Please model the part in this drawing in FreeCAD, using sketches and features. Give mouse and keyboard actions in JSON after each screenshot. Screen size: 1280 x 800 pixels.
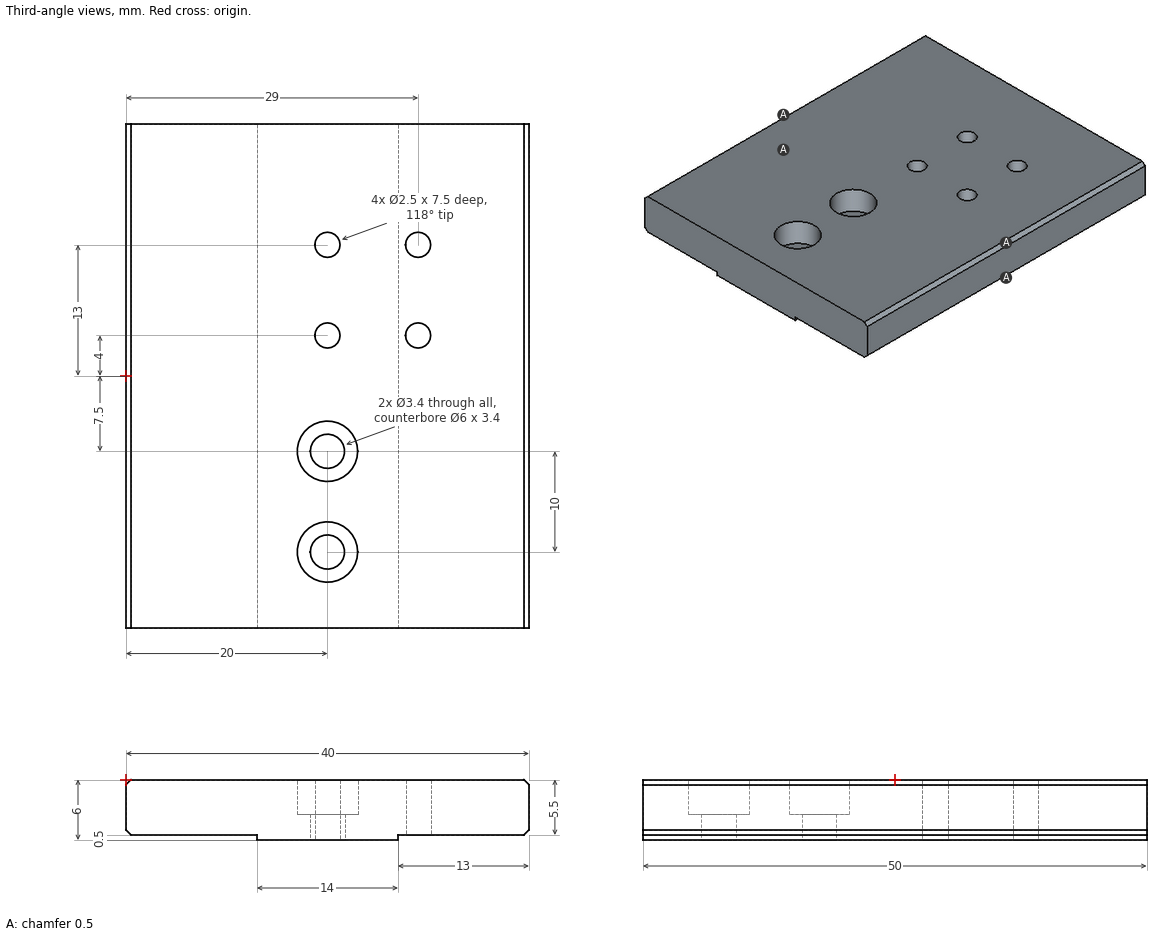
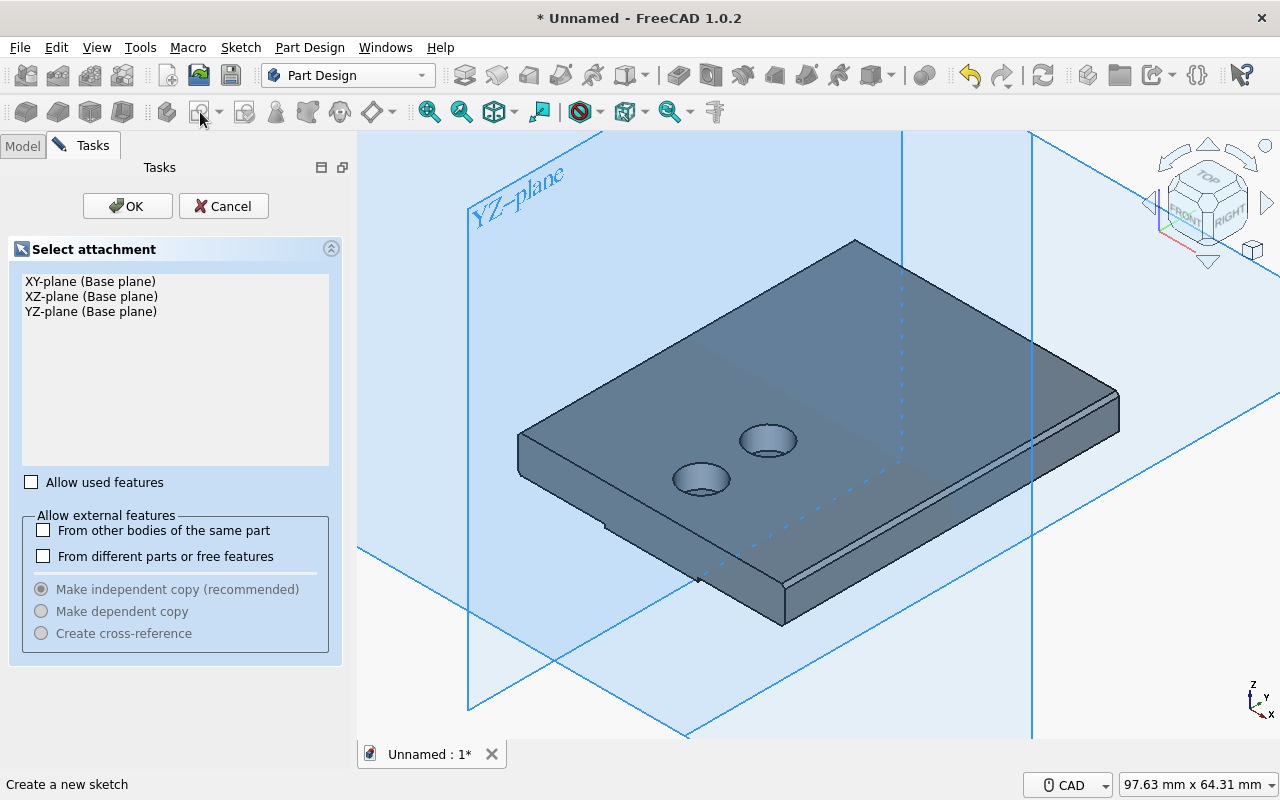
{"action": "left_click", "coordinate": [82, 282]}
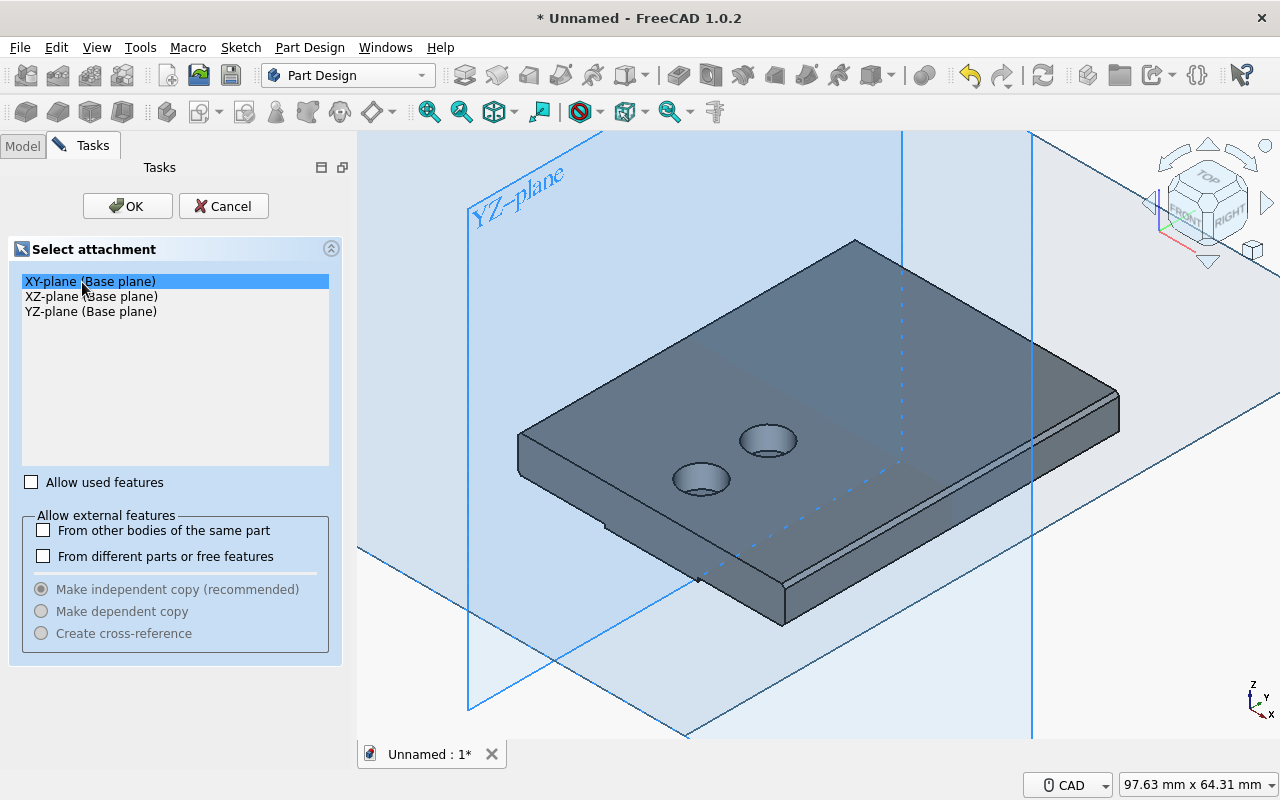
{"action": "left_click", "coordinate": [128, 206]}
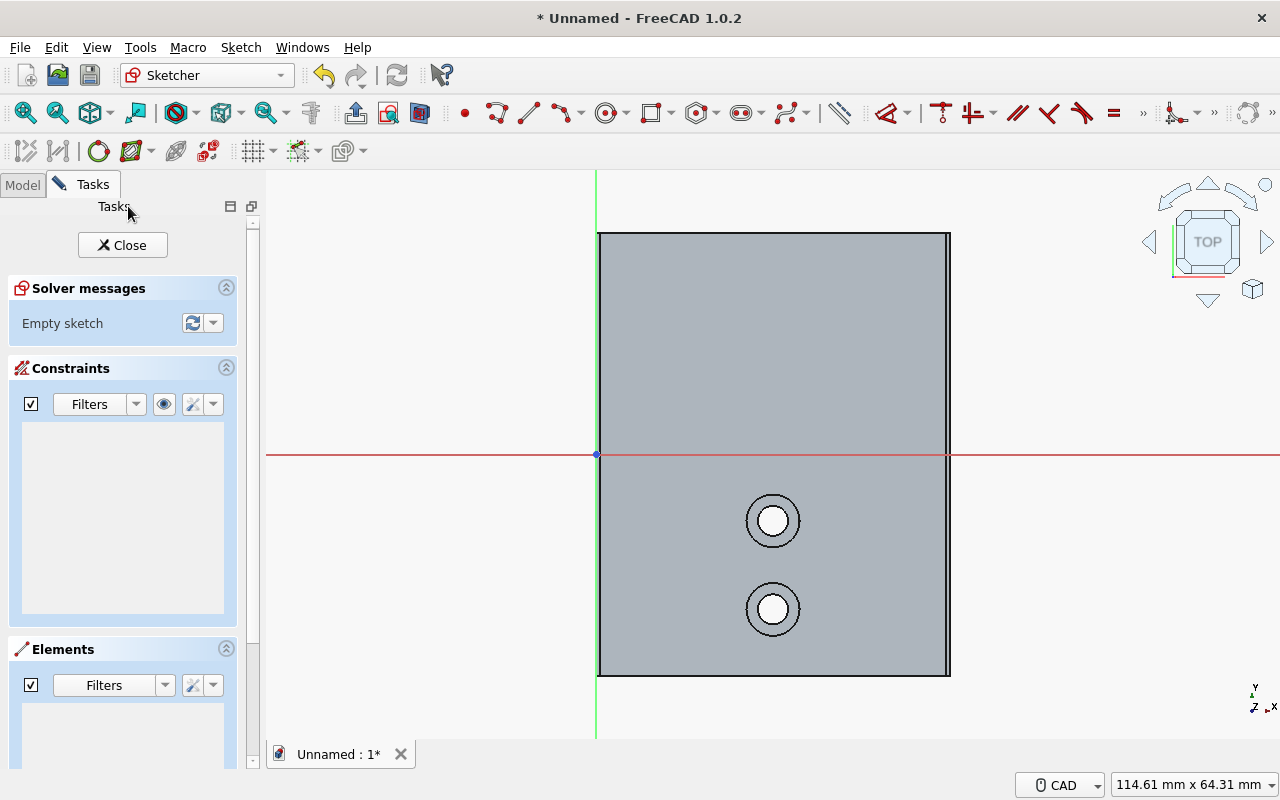
{"action": "scroll", "coordinate": [859, 347], "scroll_direction": "up", "scroll_amount": 6}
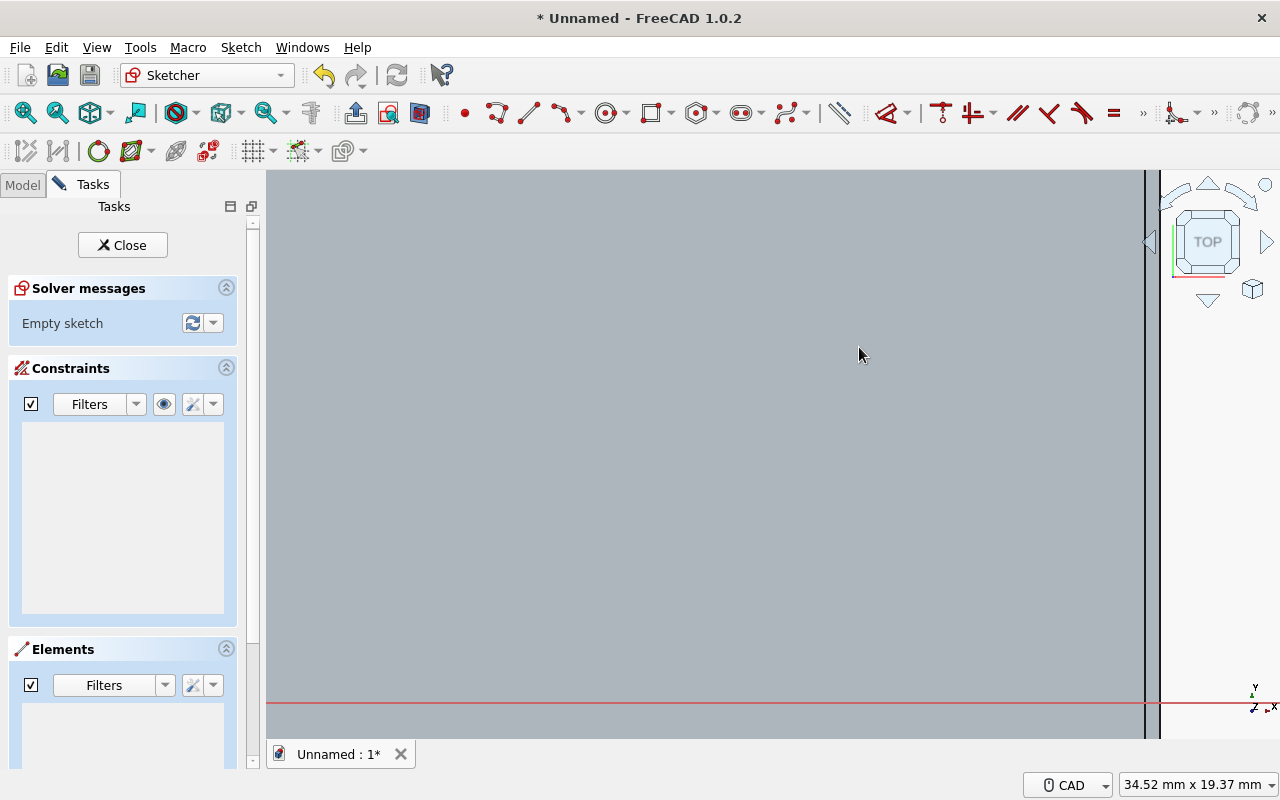
{"action": "left_click", "coordinate": [606, 114]}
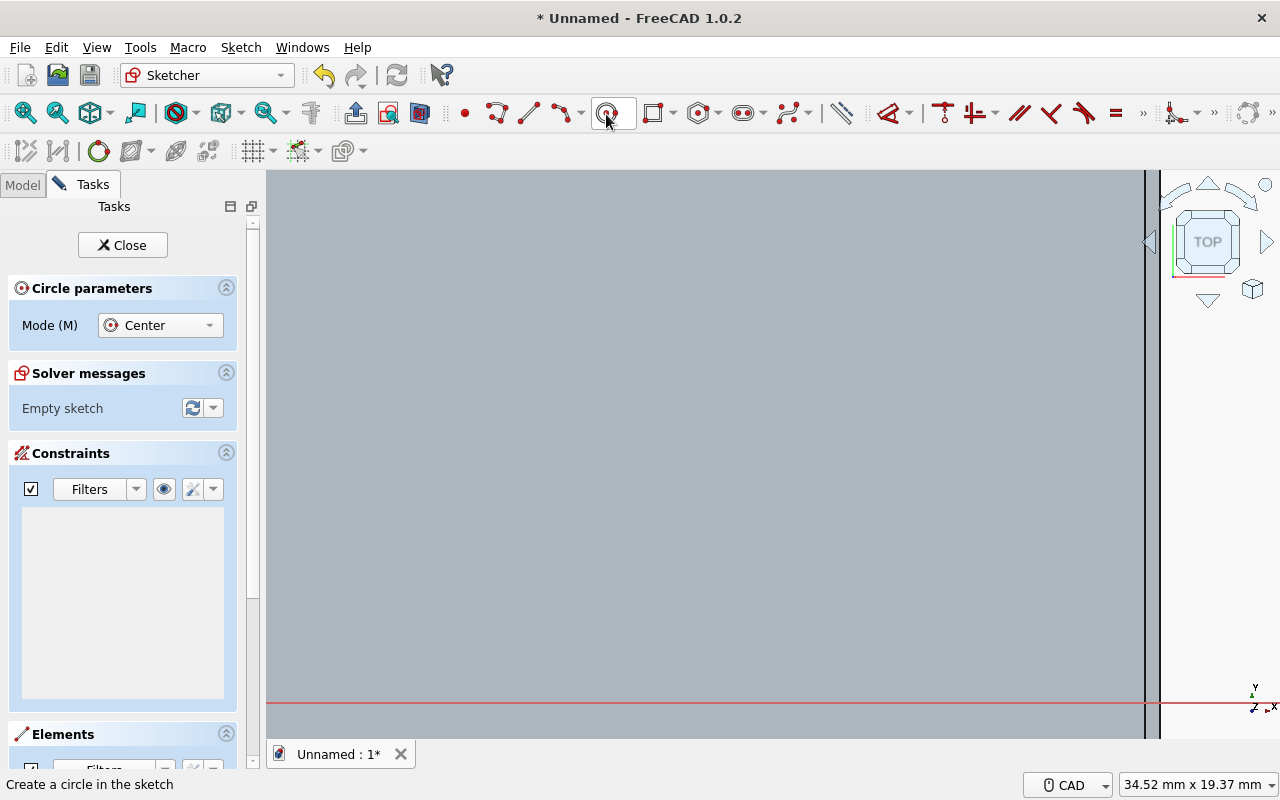
{"action": "left_click", "coordinate": [572, 321]}
{"action": "mouse_move", "coordinate": [598, 295]}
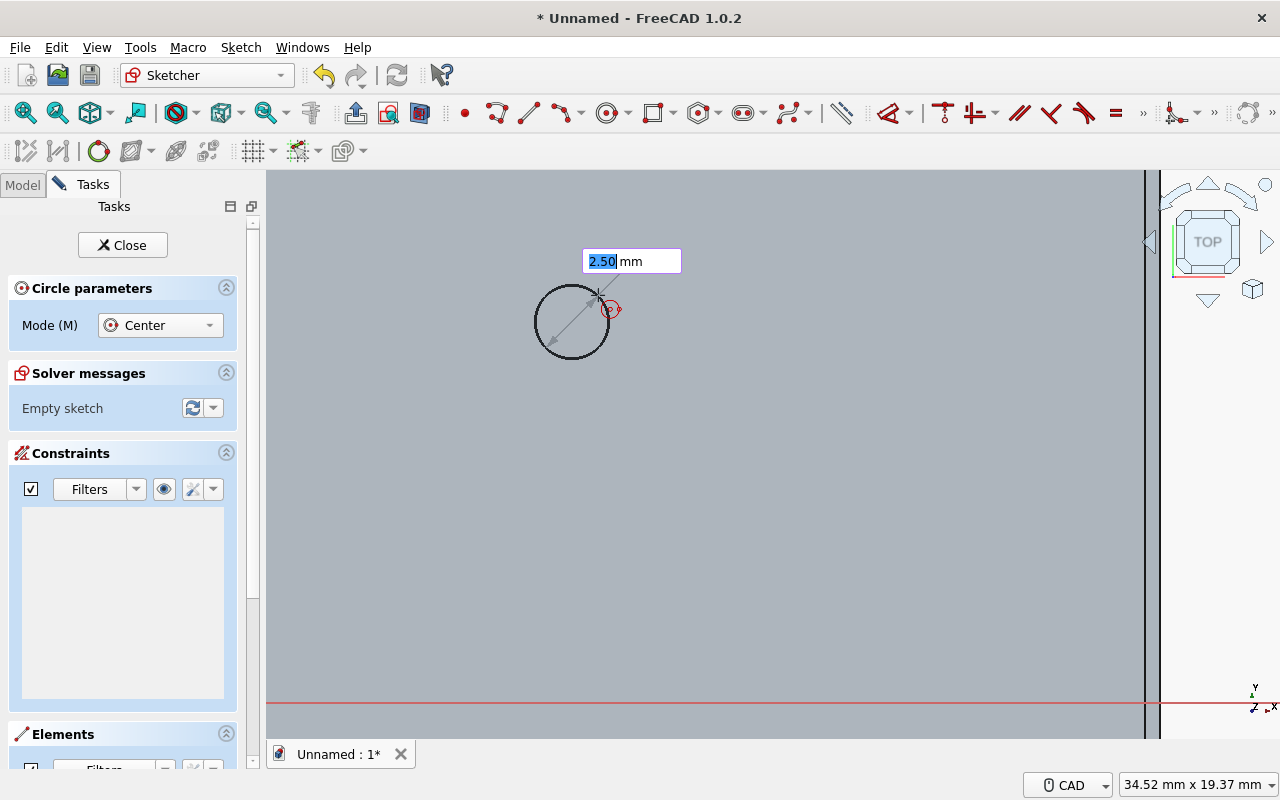
{"action": "type", "text": "2.5"}
{"action": "key", "text": "Return"}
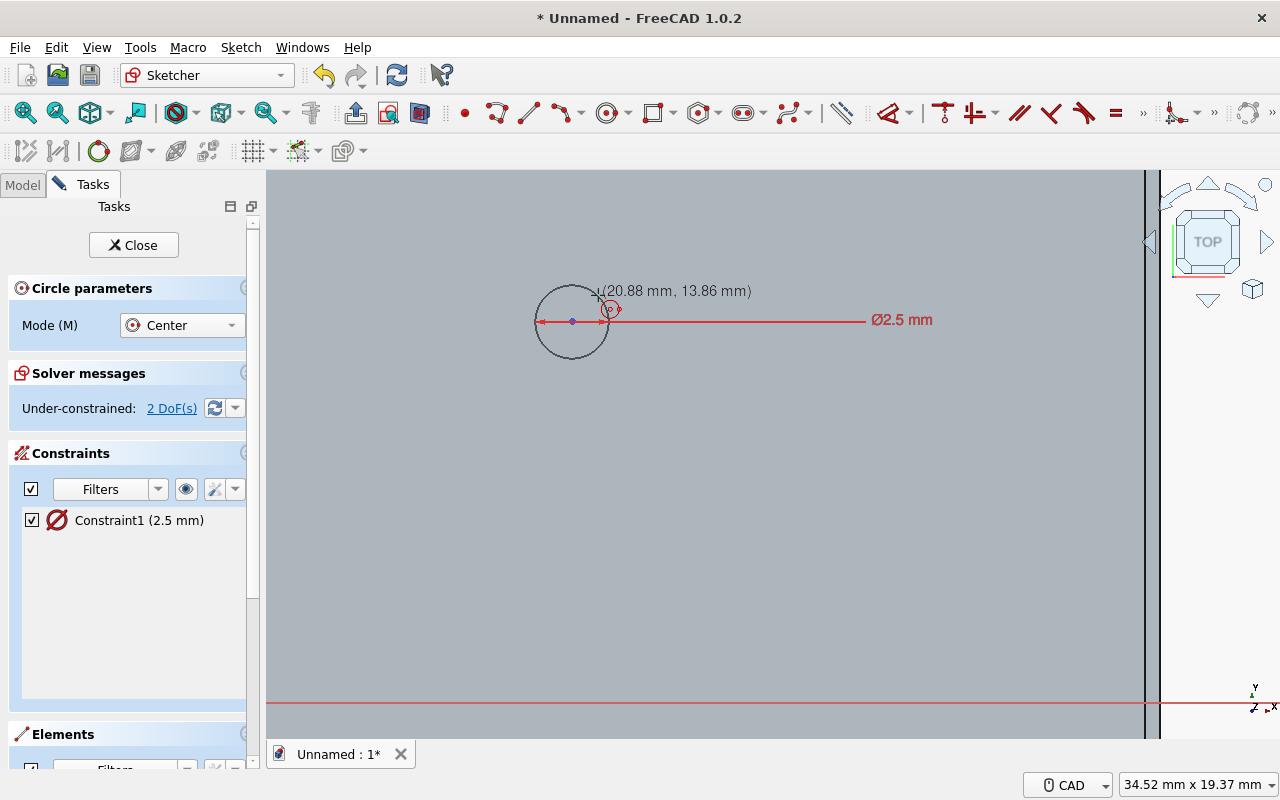
{"action": "left_click", "coordinate": [836, 321]}
{"action": "mouse_move", "coordinate": [862, 295]}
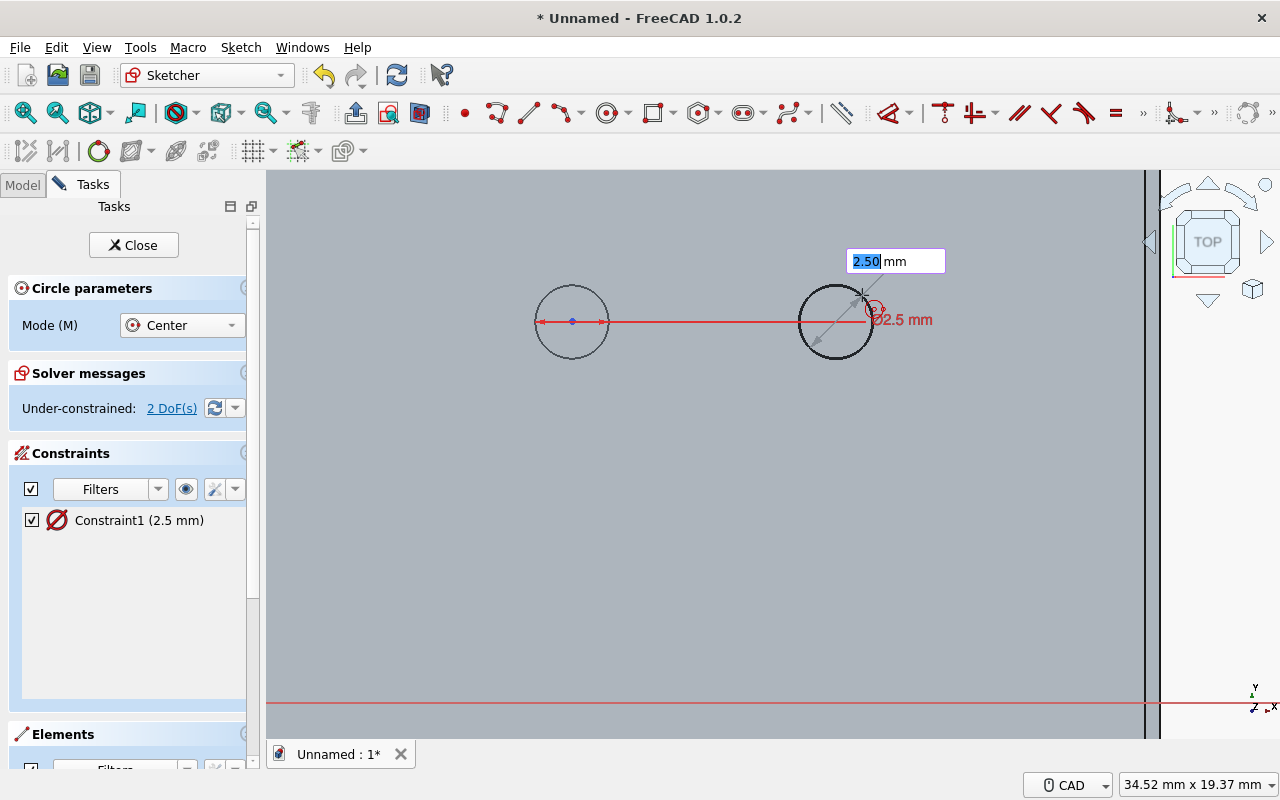
{"action": "type", "text": "2.5"}
{"action": "key", "text": "Return"}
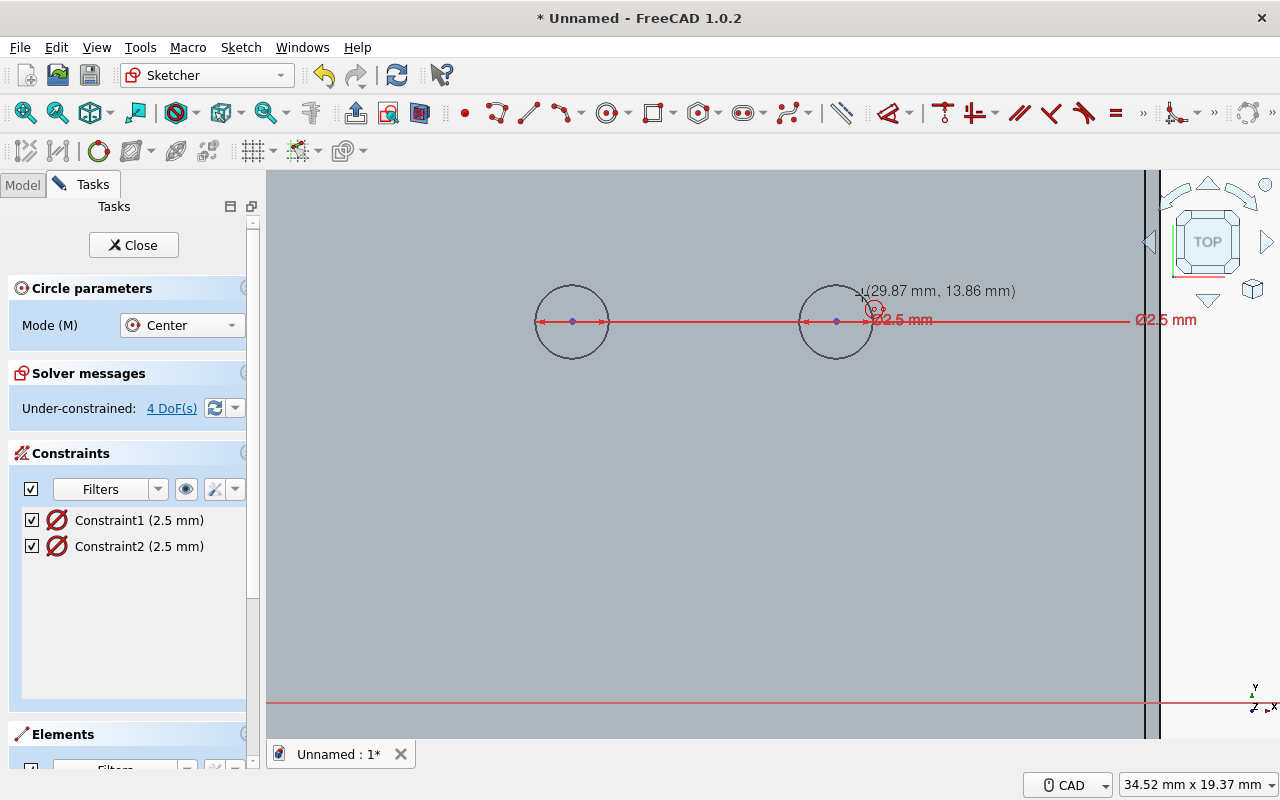
{"action": "left_click", "coordinate": [572, 586]}
{"action": "mouse_move", "coordinate": [598, 560]}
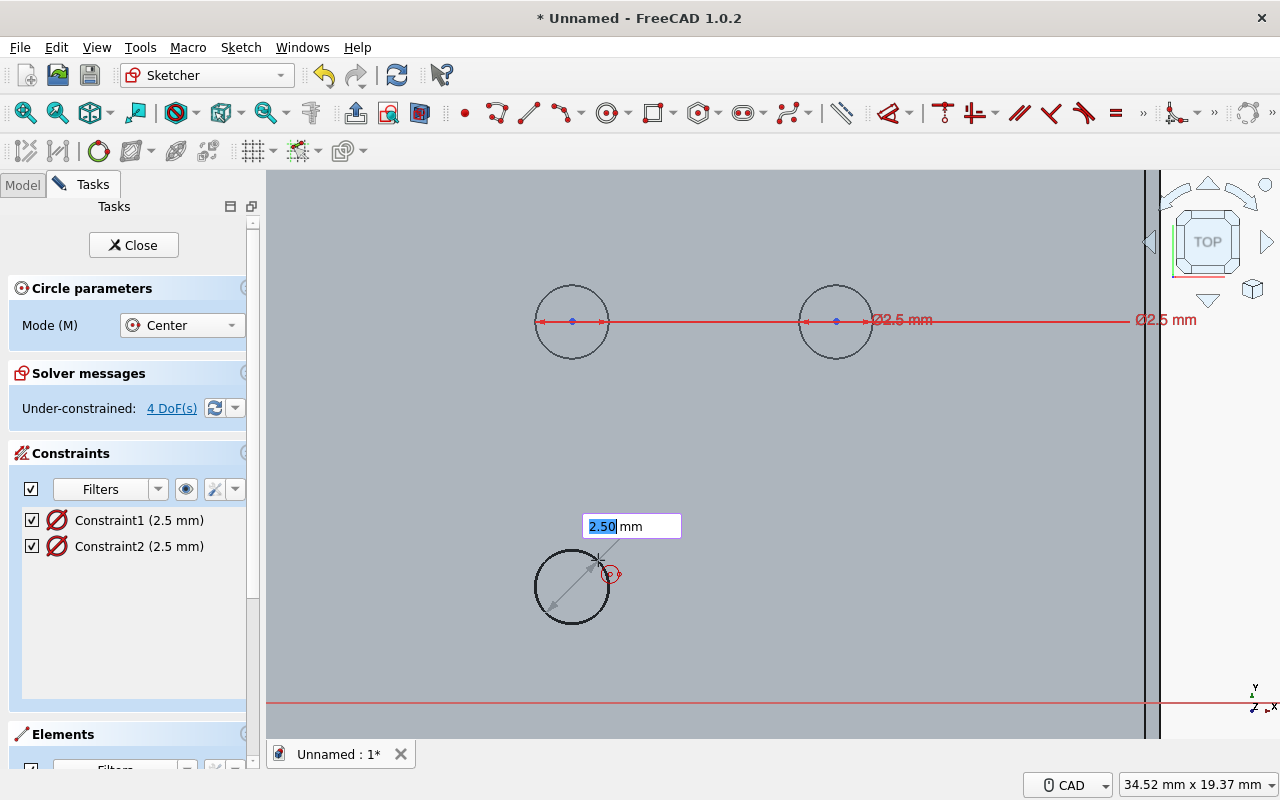
{"action": "type", "text": "2.5"}
{"action": "key", "text": "Return"}